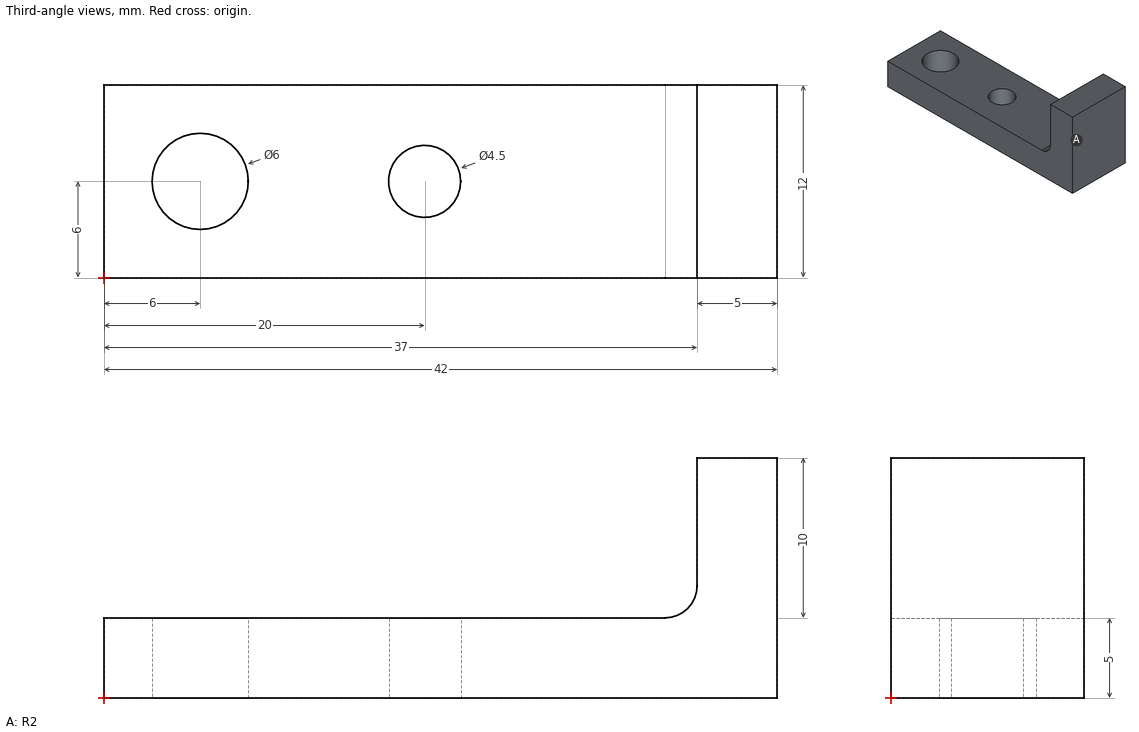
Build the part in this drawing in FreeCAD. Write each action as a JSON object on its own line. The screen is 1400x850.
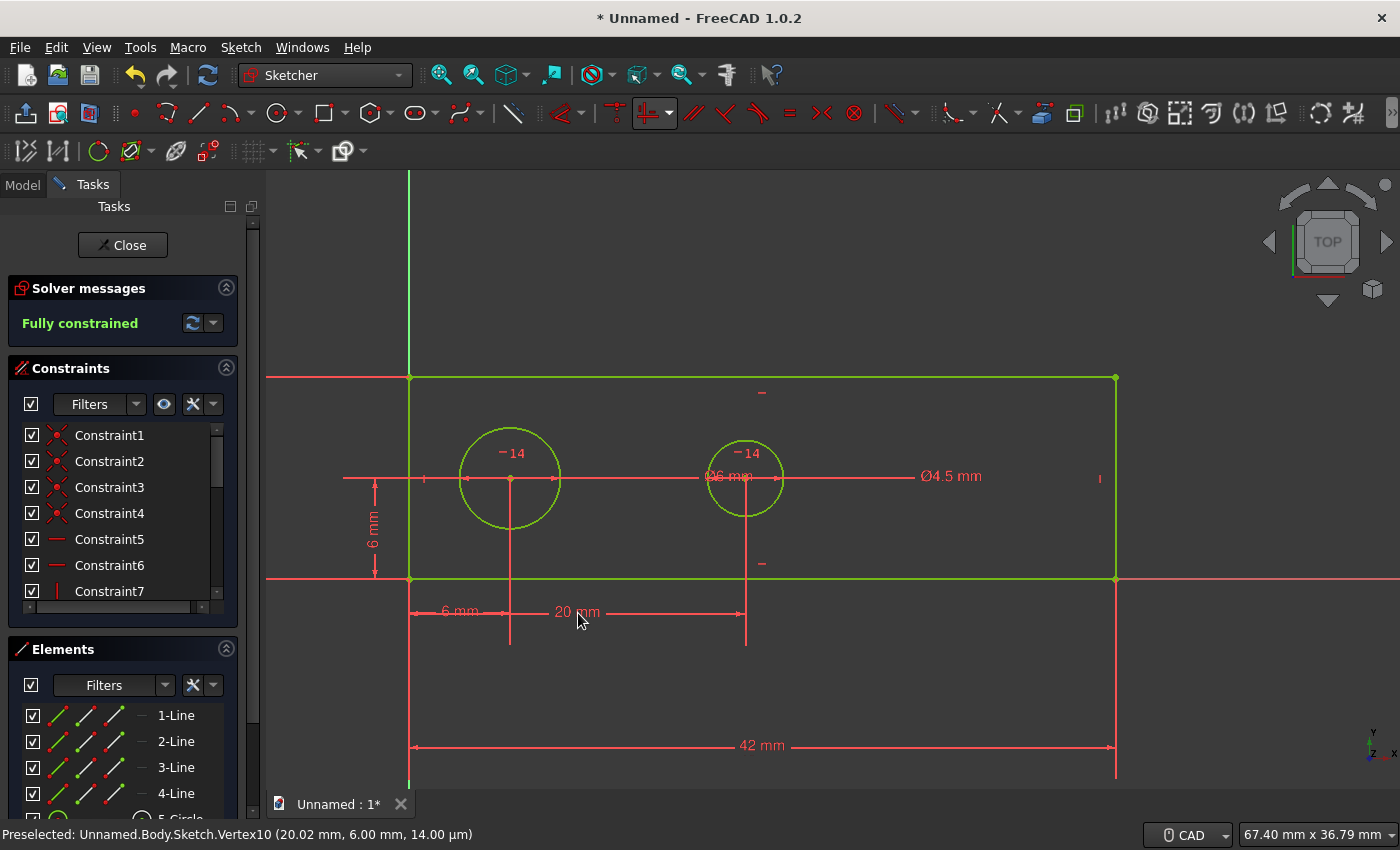
{"action": "left_click", "coordinate": [123, 245]}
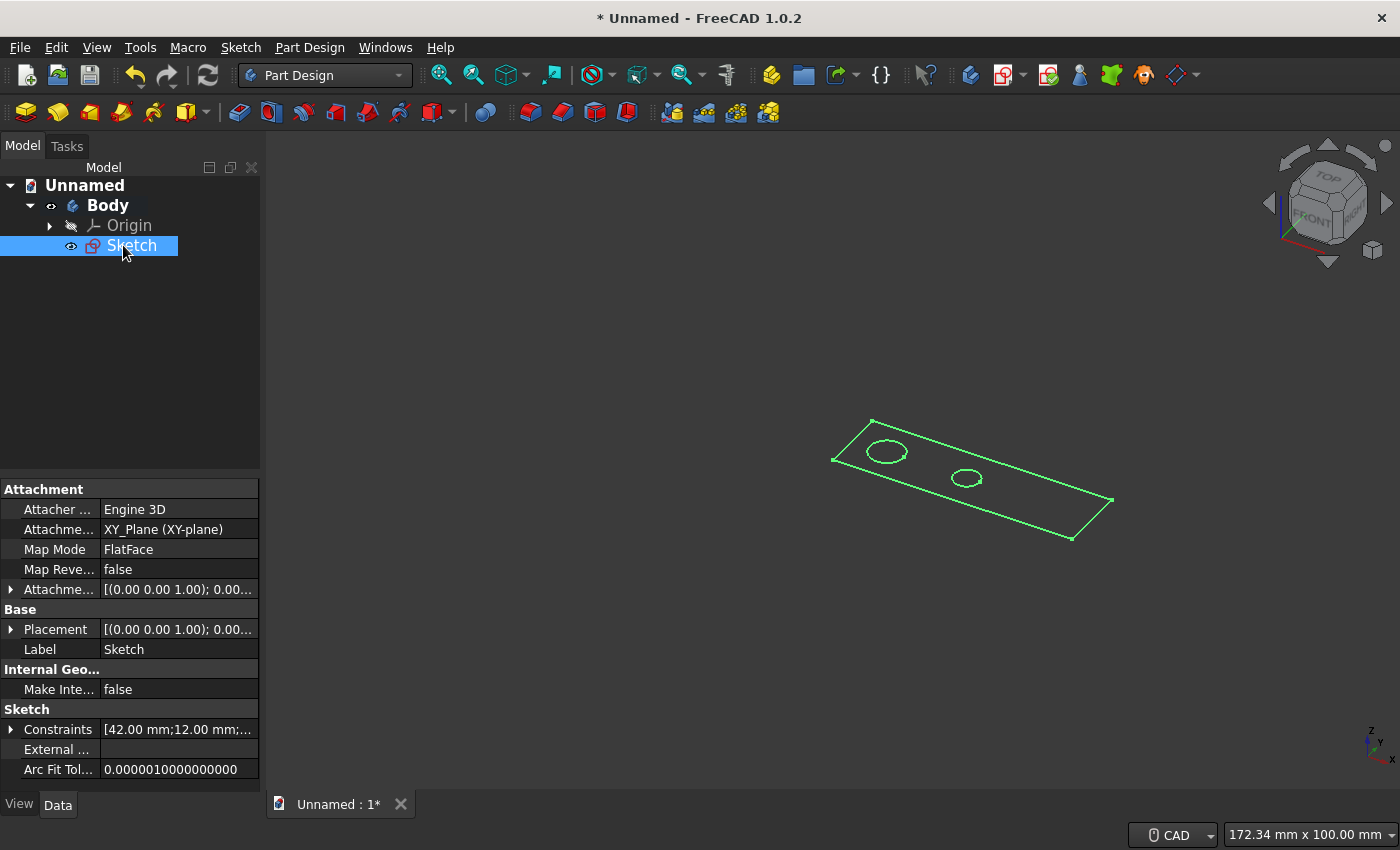
{"action": "left_click", "coordinate": [26, 112]}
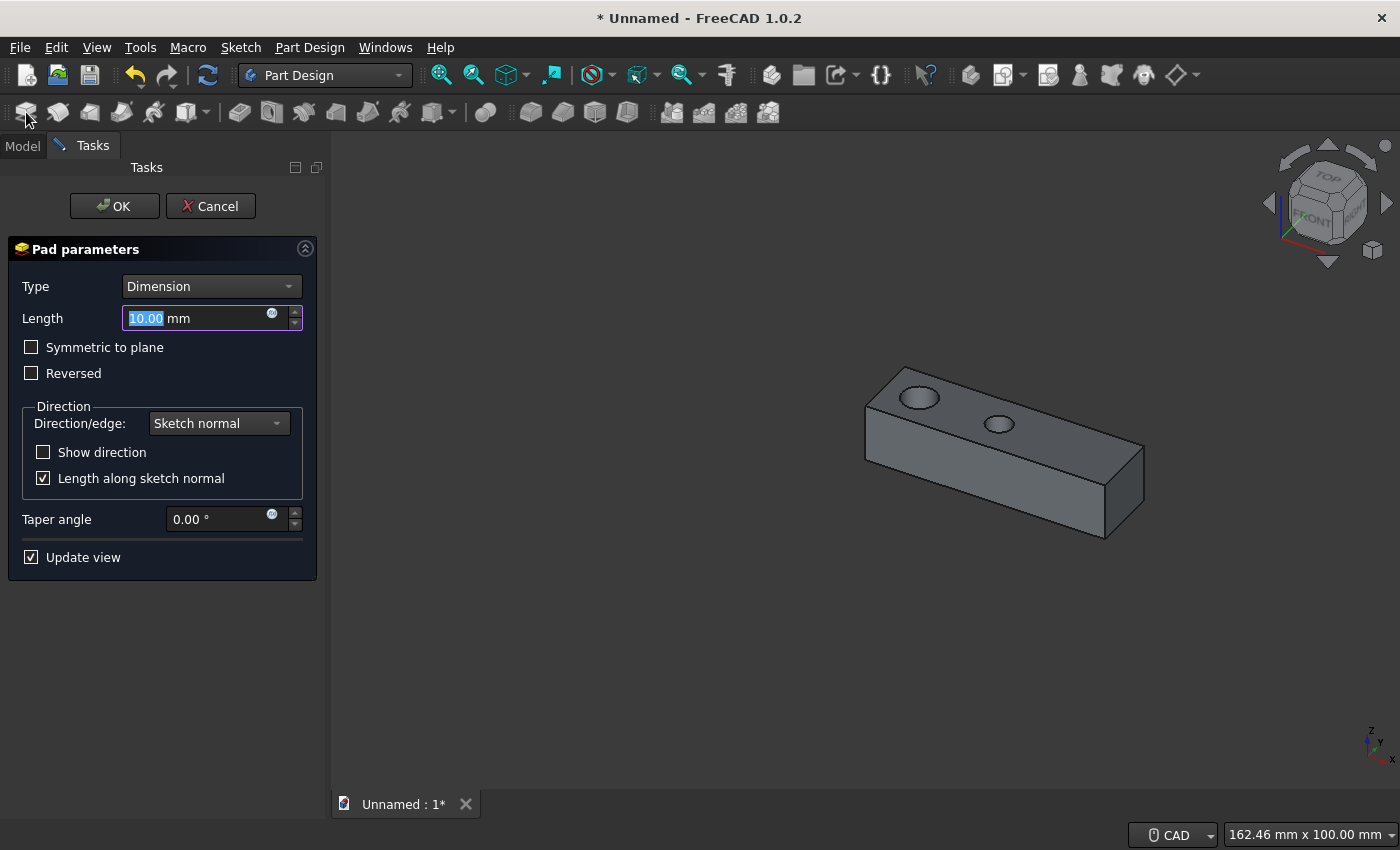
{"action": "type", "text": "5"}
{"action": "key", "text": "Tab"}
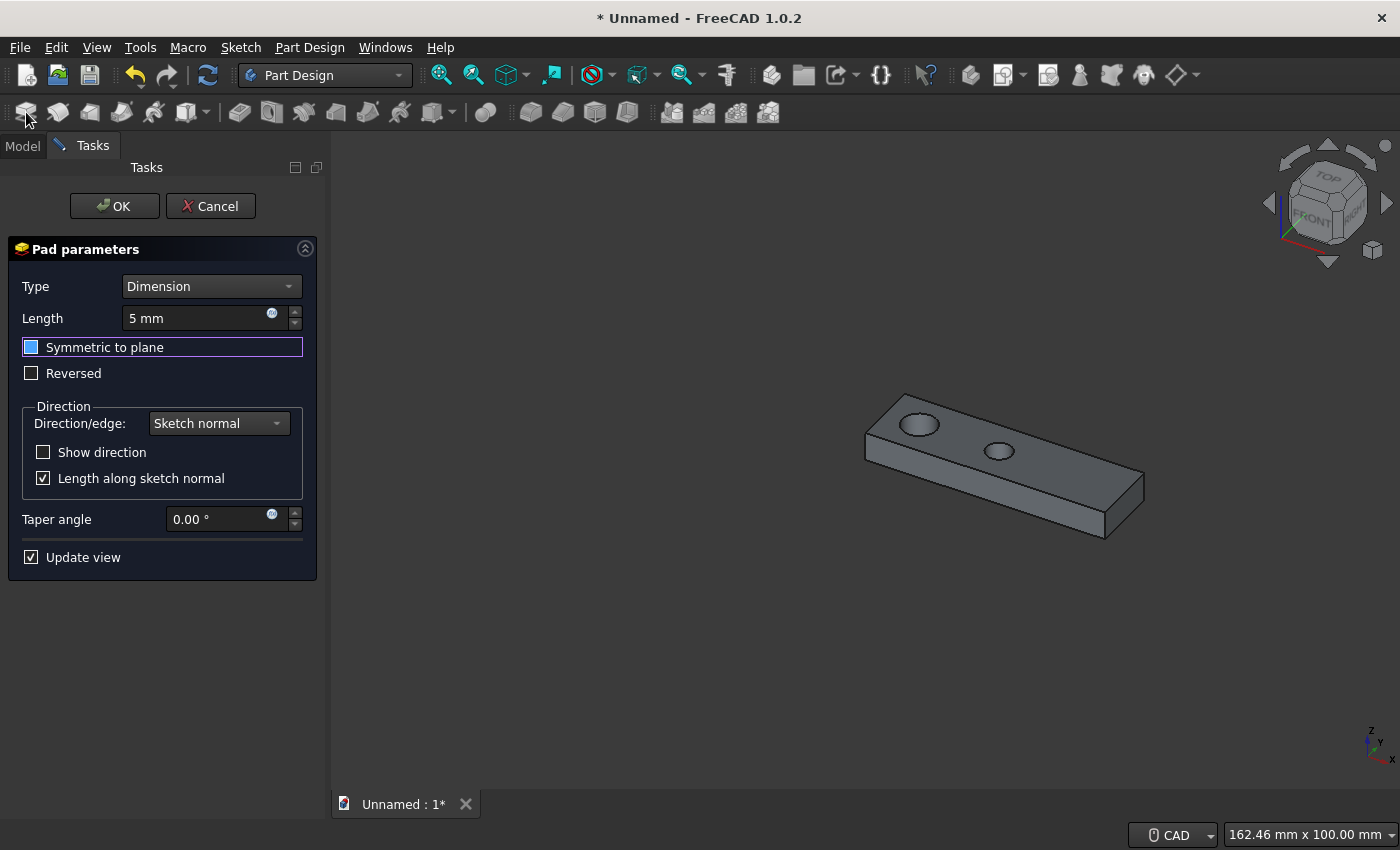
{"action": "left_click", "coordinate": [115, 206]}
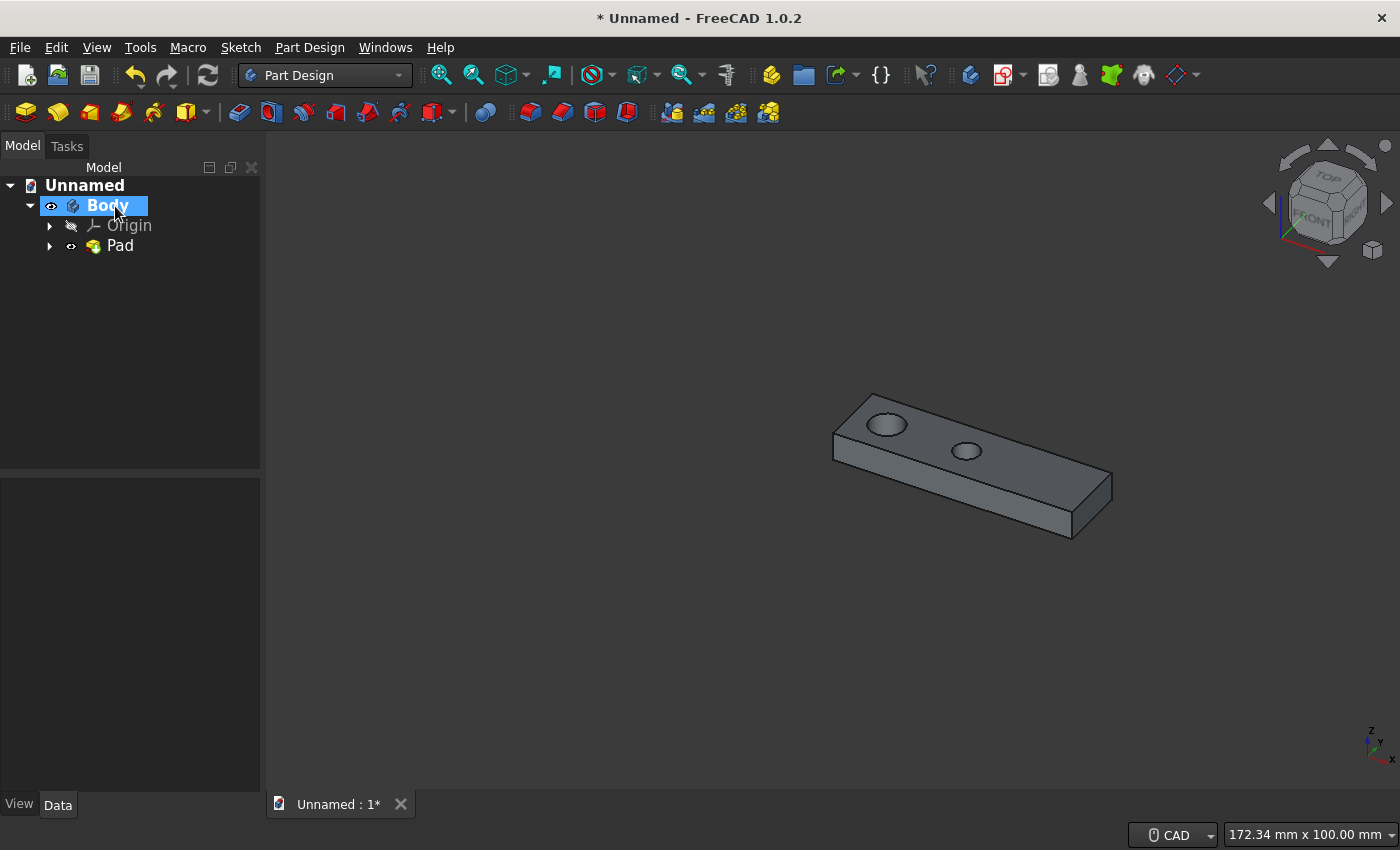
{"action": "left_click", "coordinate": [442, 76]}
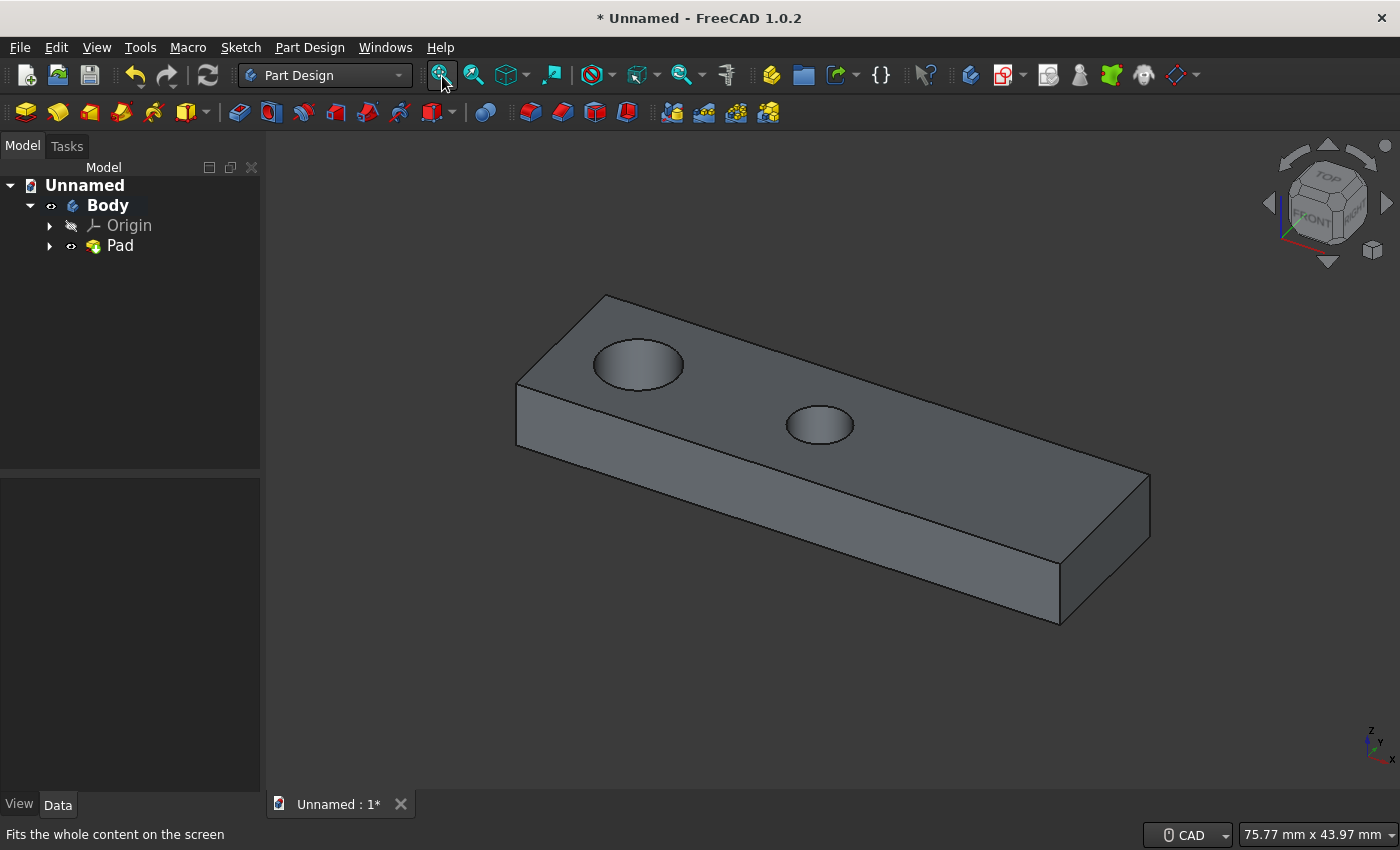
{"action": "left_click", "coordinate": [989, 480]}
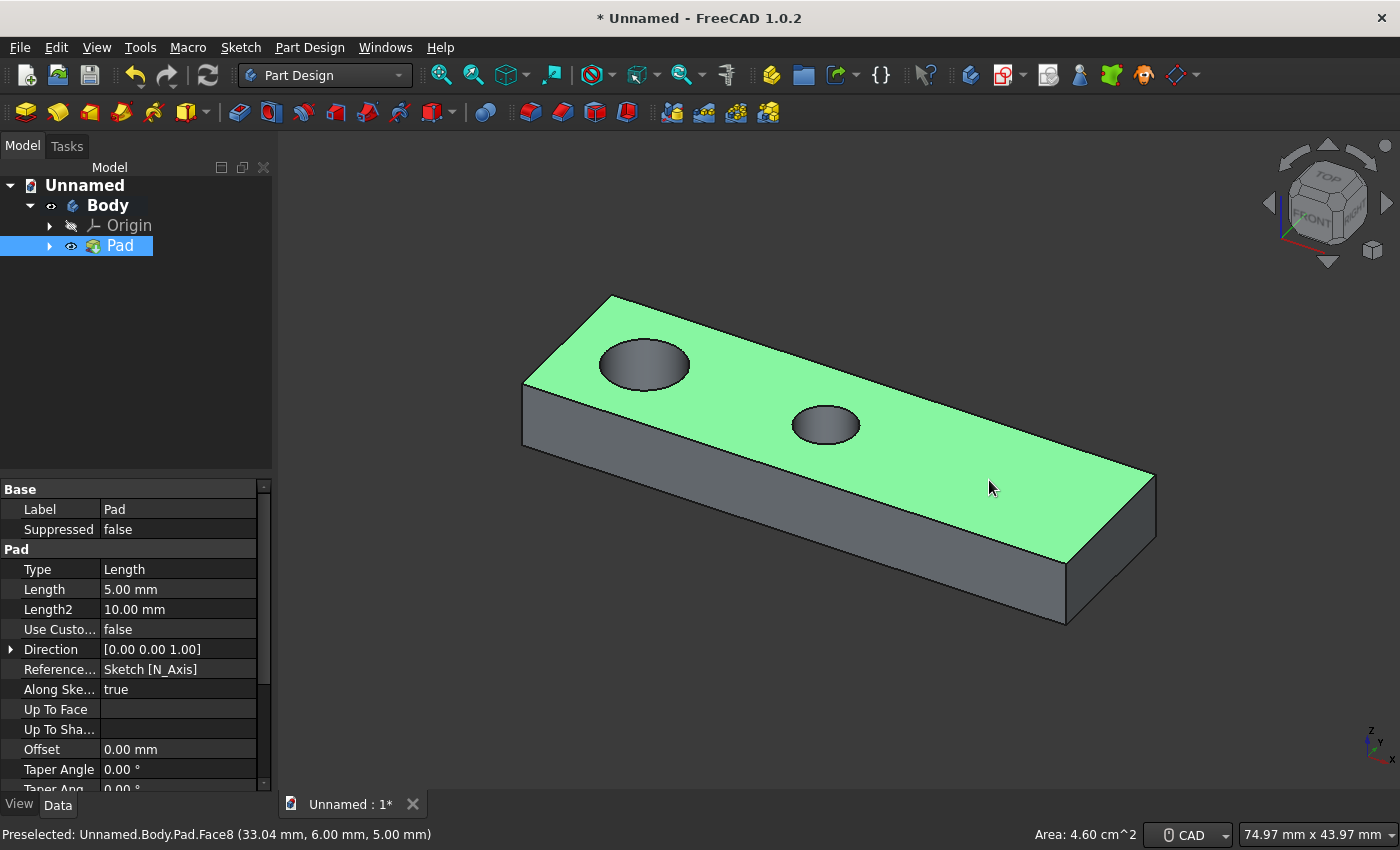
{"action": "left_click", "coordinate": [1004, 76]}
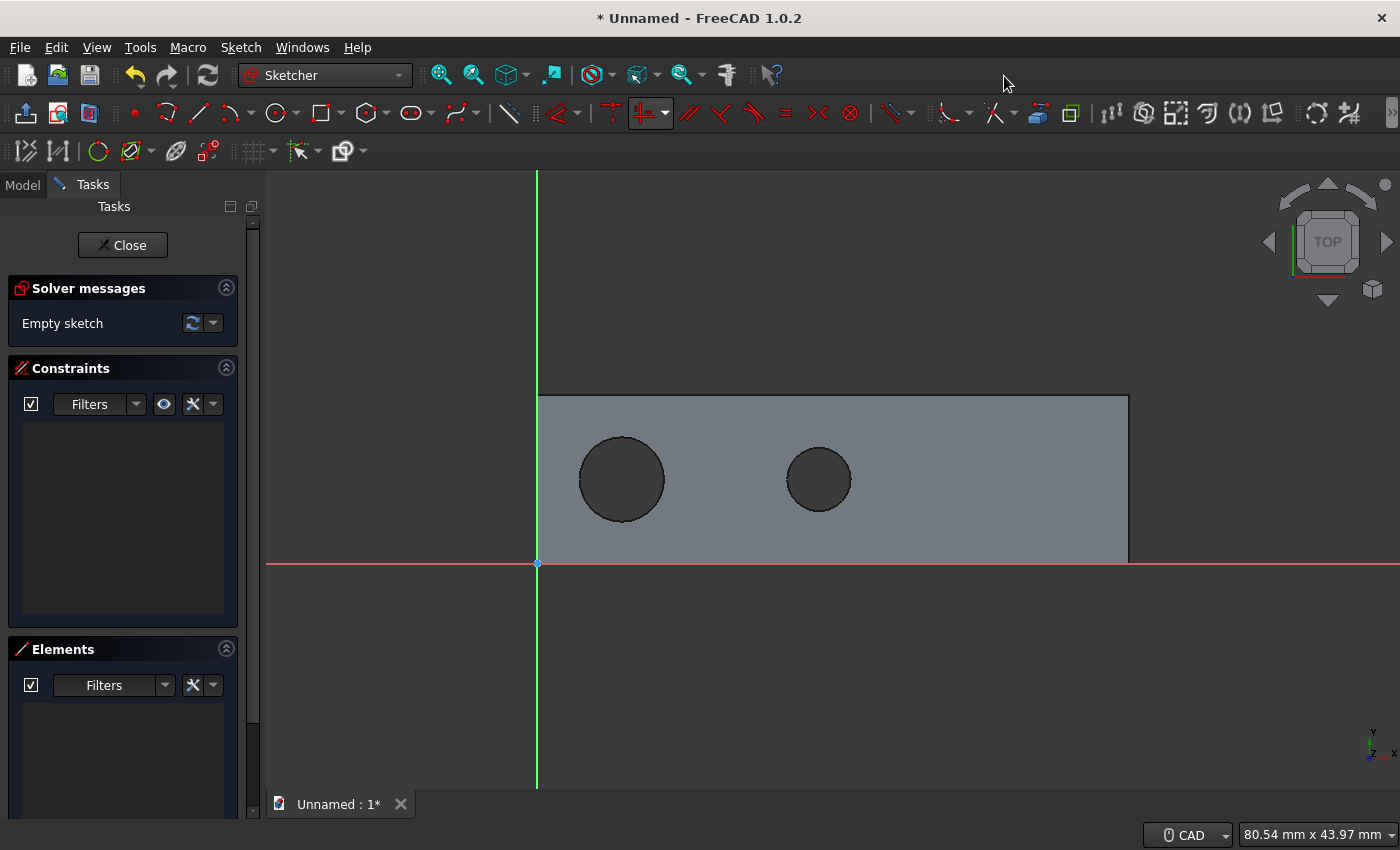
{"action": "scroll", "coordinate": [1235, 480], "scroll_direction": "up", "scroll_amount": 4}